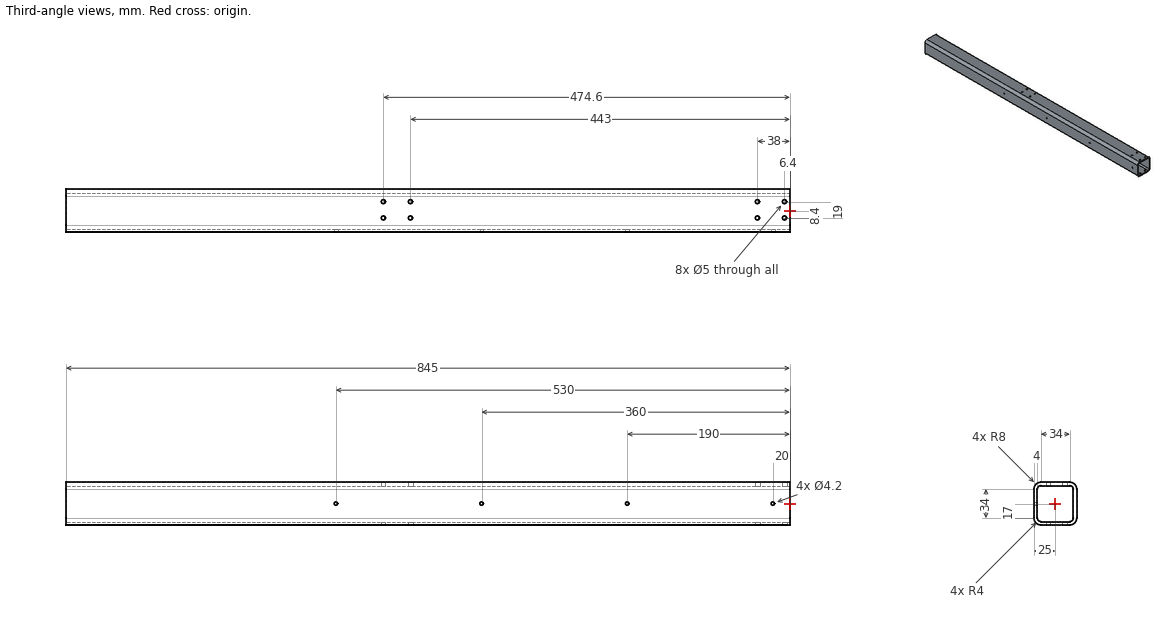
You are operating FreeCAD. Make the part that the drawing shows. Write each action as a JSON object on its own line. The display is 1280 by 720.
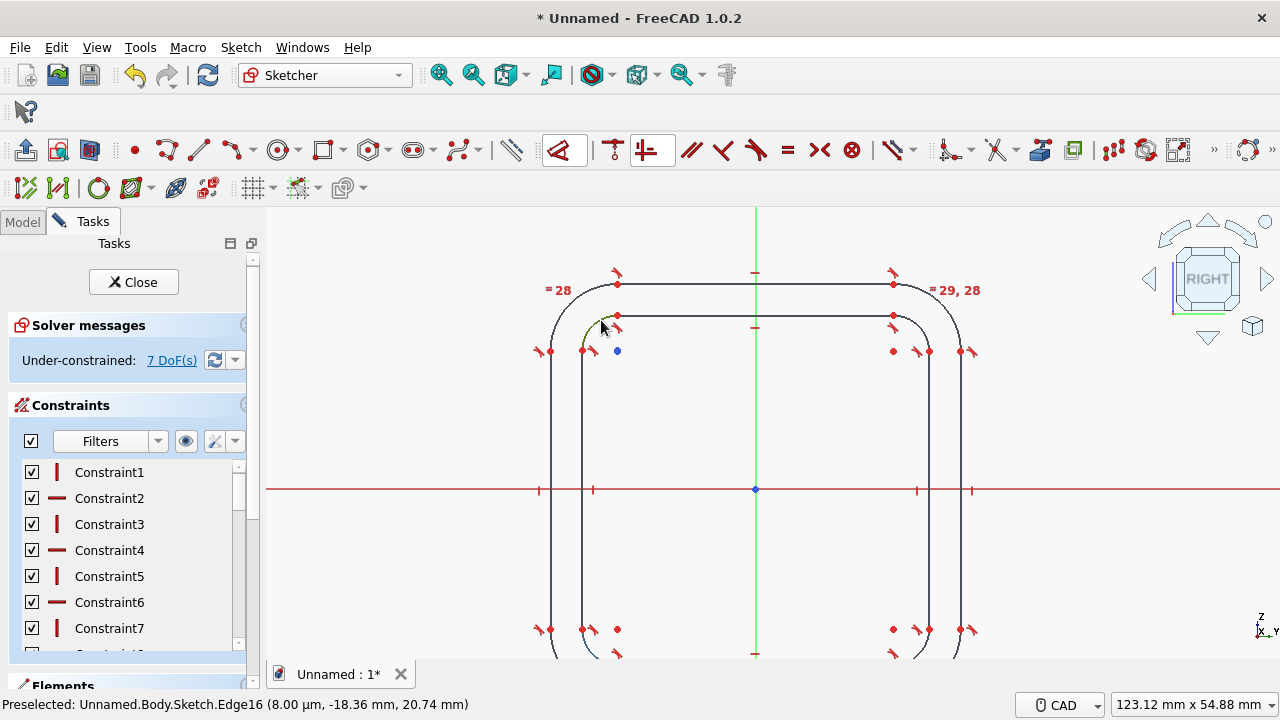
{"action": "left_click", "coordinate": [788, 150]}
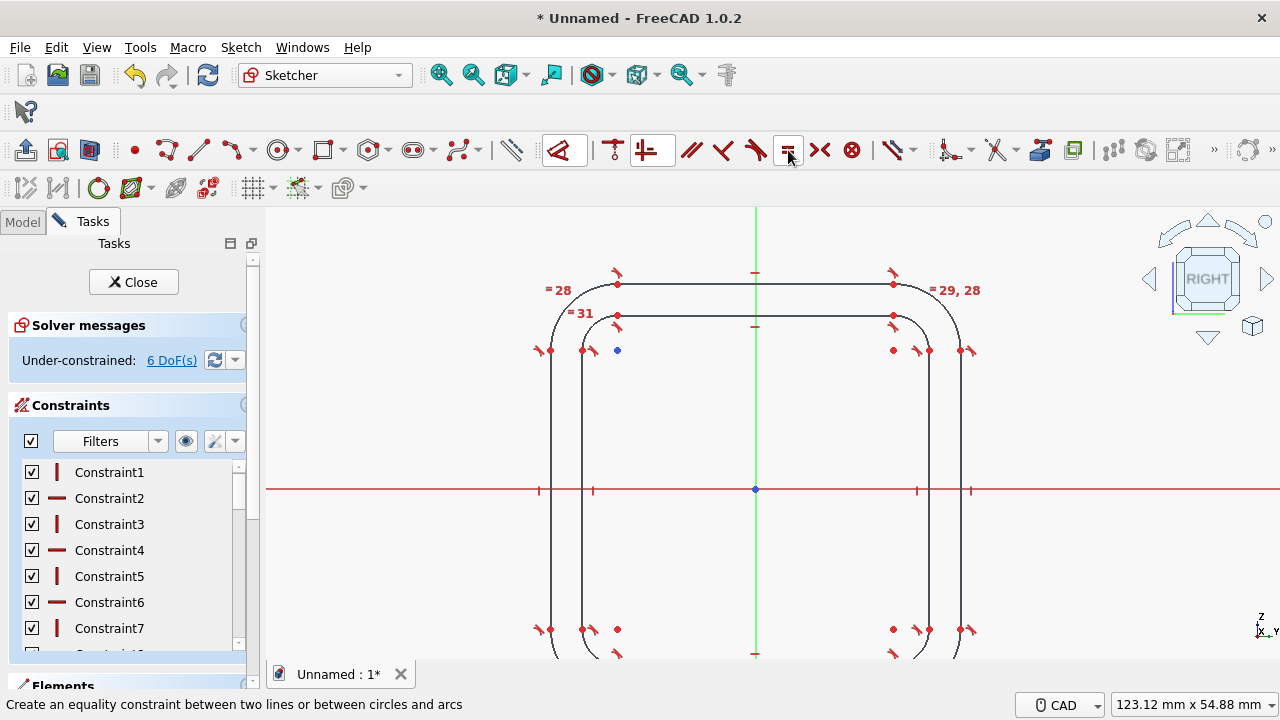
{"action": "left_click", "coordinate": [587, 291]}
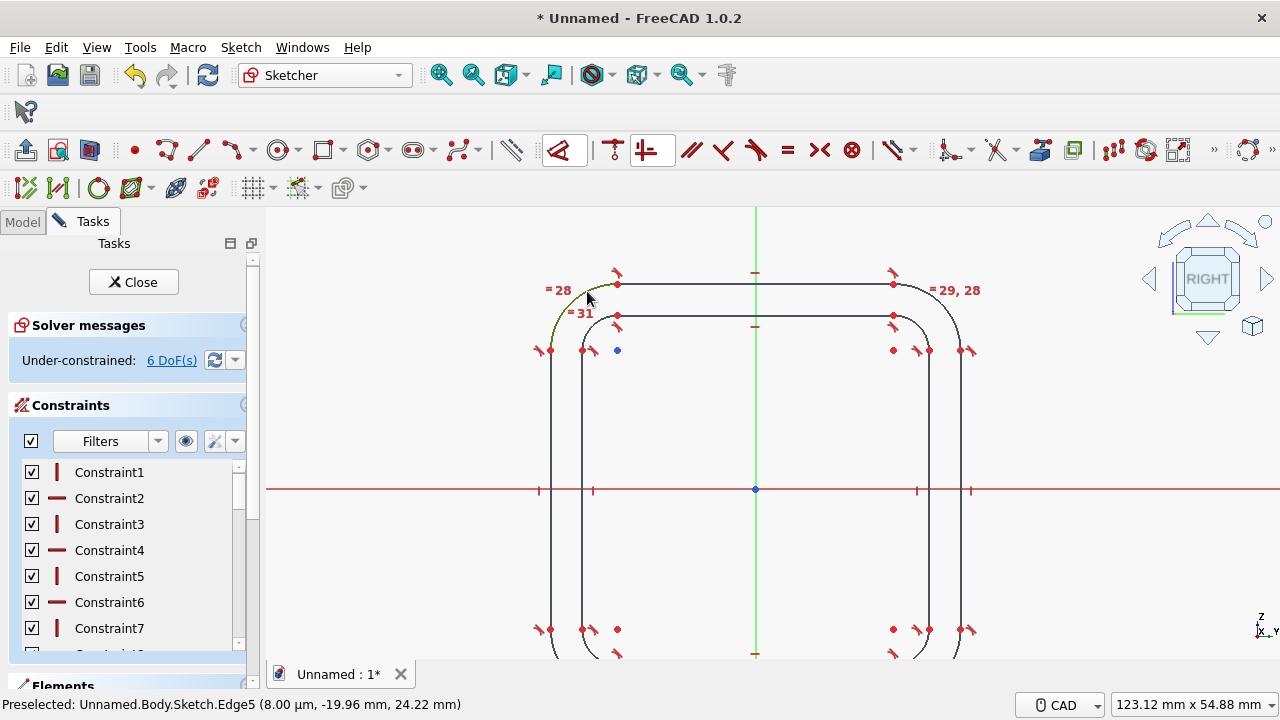
{"action": "key", "text": "k r"}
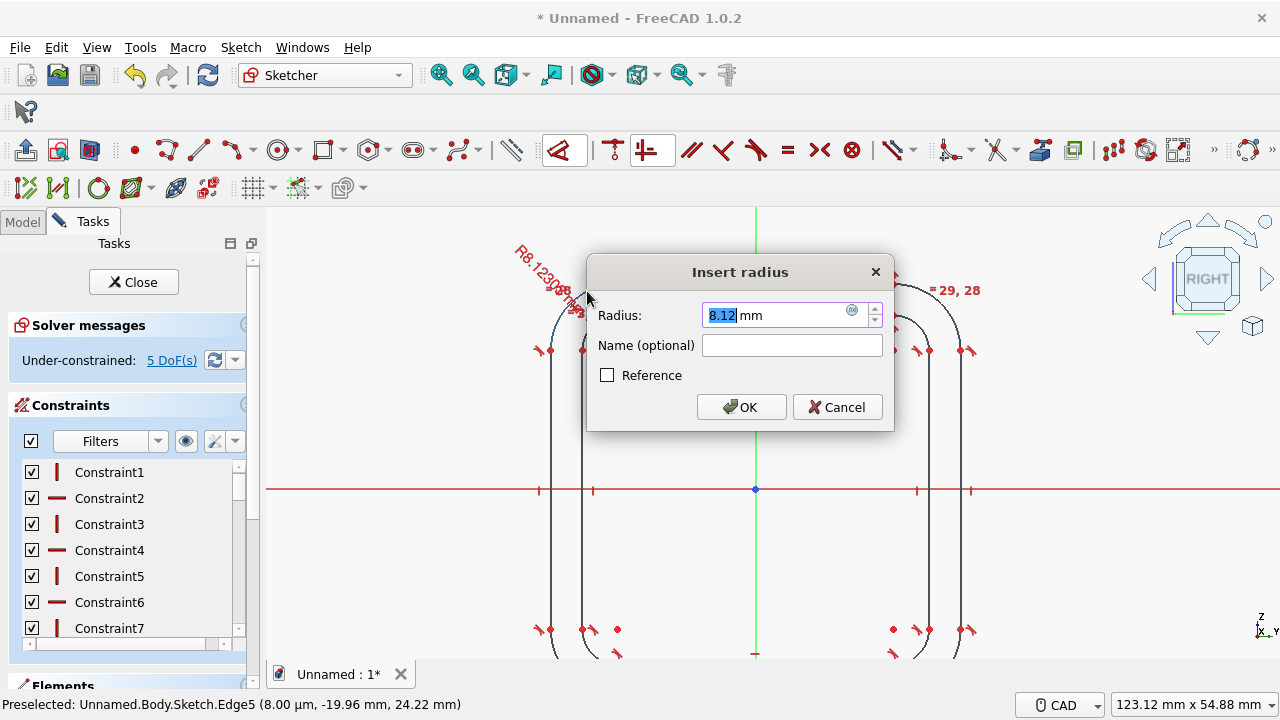
{"action": "type", "text": "8"}
{"action": "key", "text": "Return"}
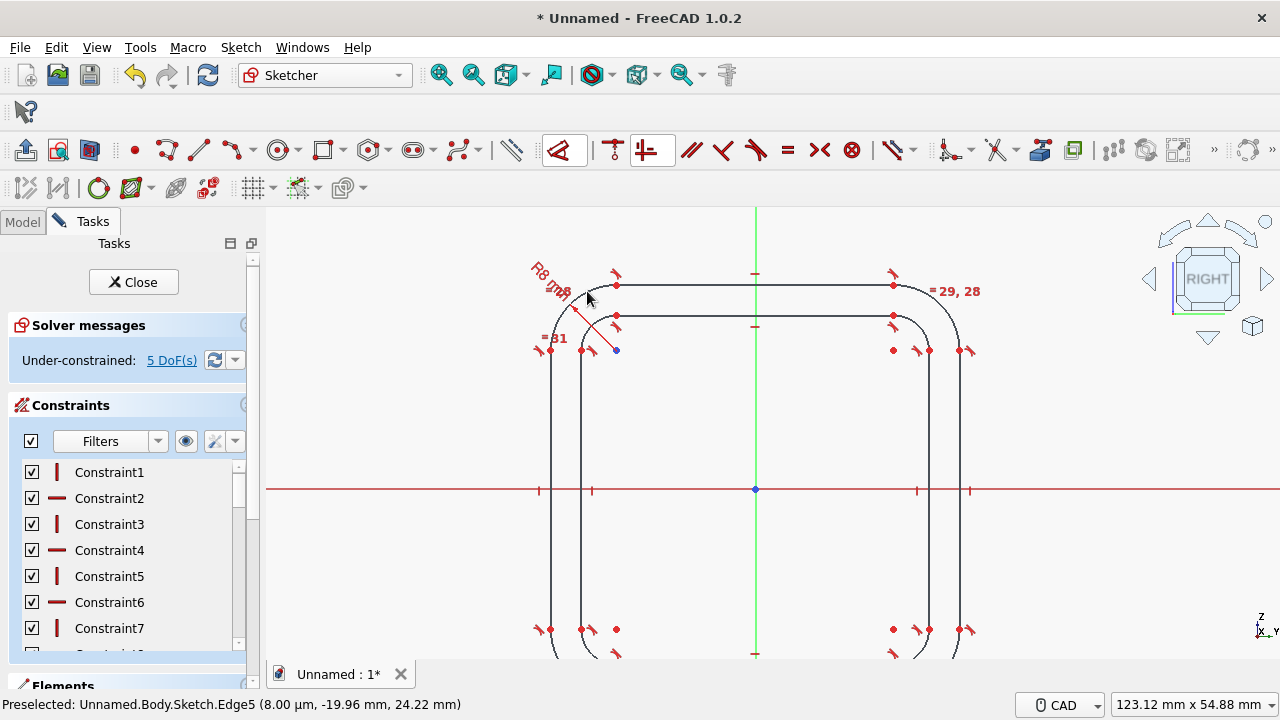
{"action": "scroll", "coordinate": [601, 319], "scroll_direction": "down", "scroll_amount": 2}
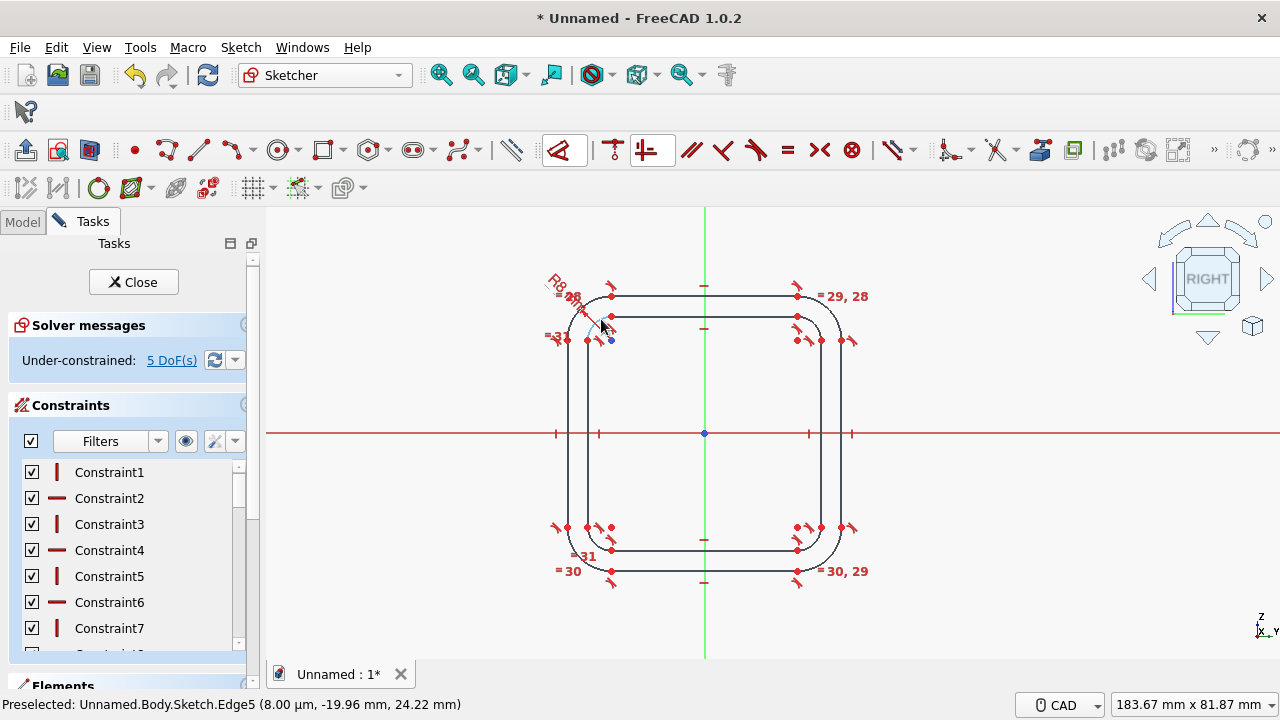
{"action": "scroll", "coordinate": [591, 538], "scroll_direction": "up", "scroll_amount": 3}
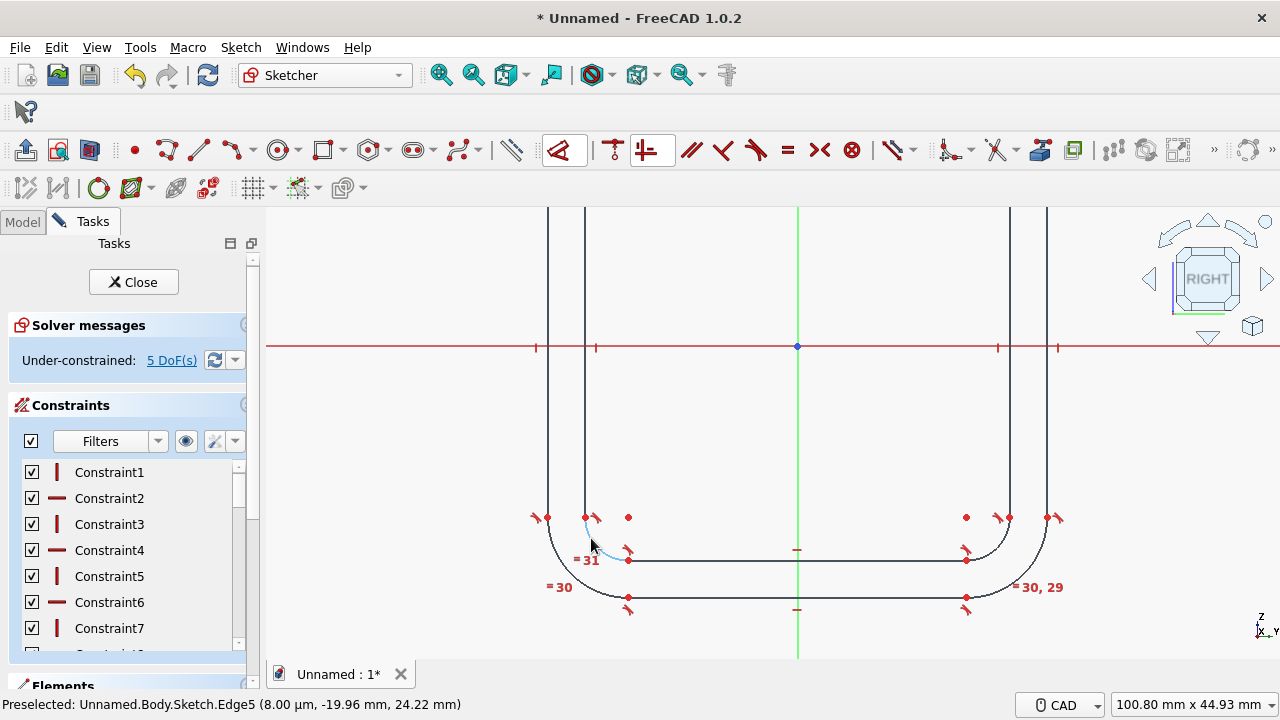
{"action": "left_click", "coordinate": [590, 537]}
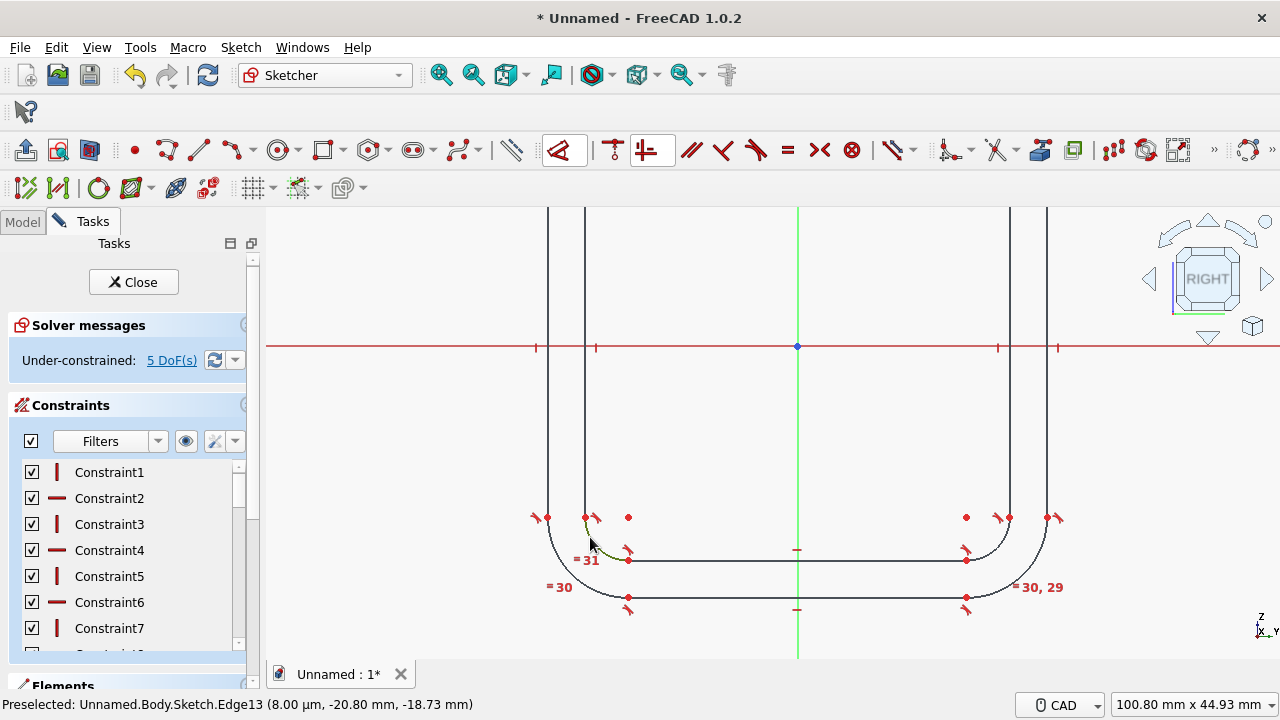
{"action": "left_click", "coordinate": [582, 150]}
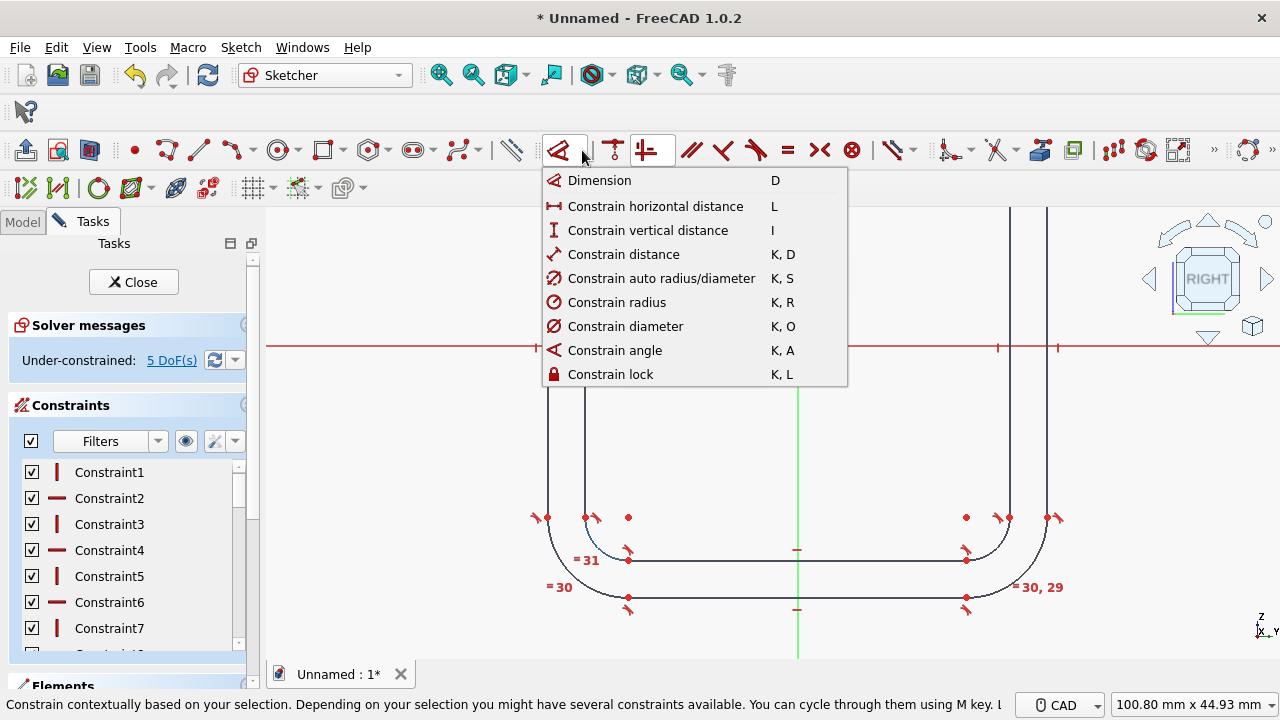
{"action": "left_click", "coordinate": [695, 302]}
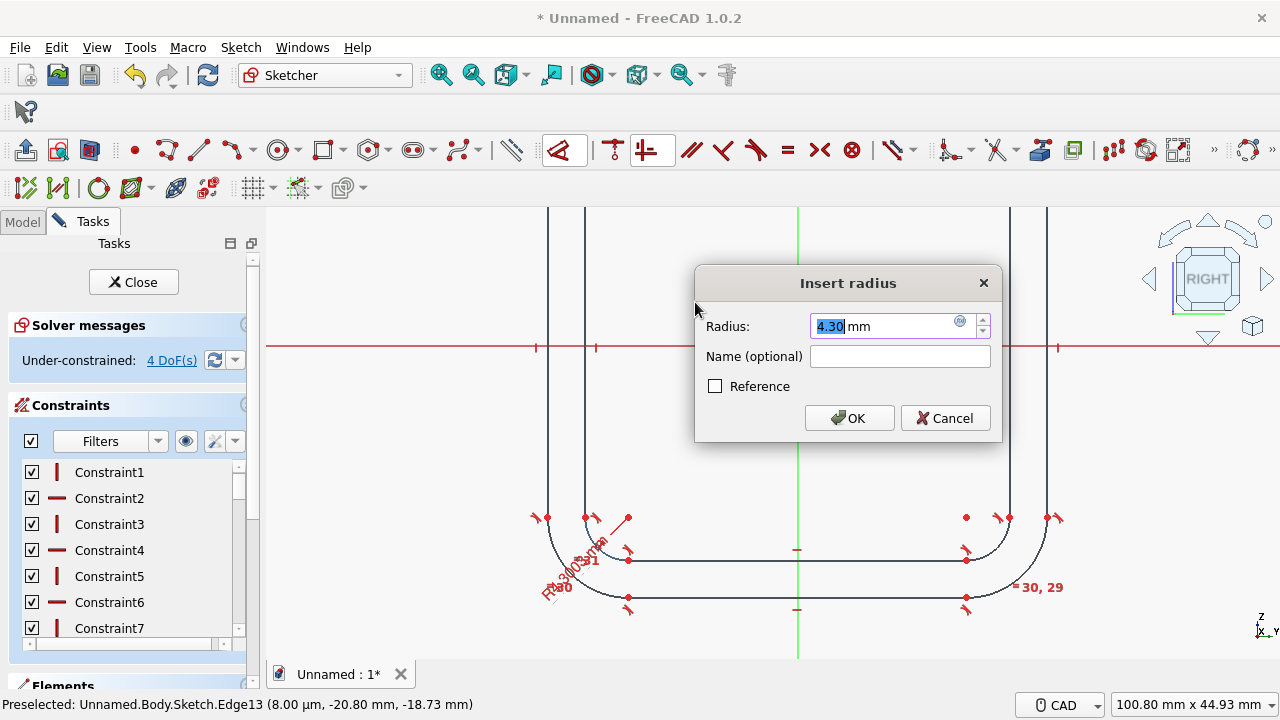
{"action": "type", "text": "4"}
{"action": "key", "text": "Return"}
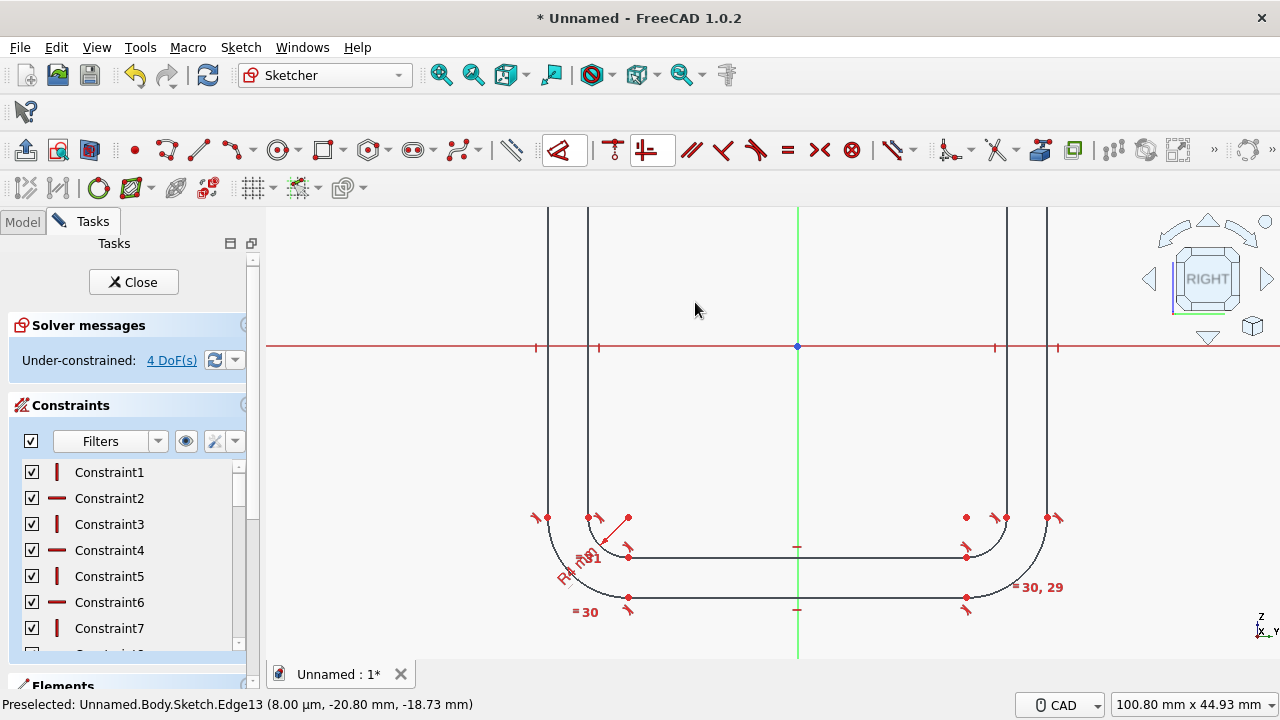
{"action": "left_click", "coordinate": [548, 415]}